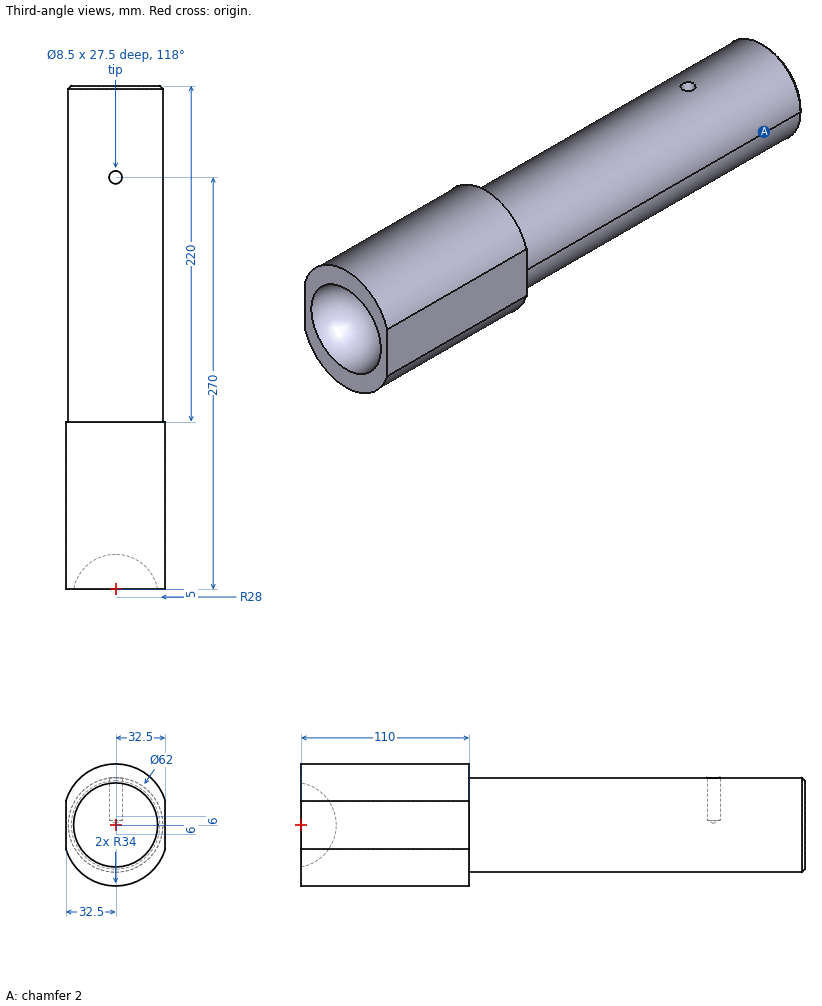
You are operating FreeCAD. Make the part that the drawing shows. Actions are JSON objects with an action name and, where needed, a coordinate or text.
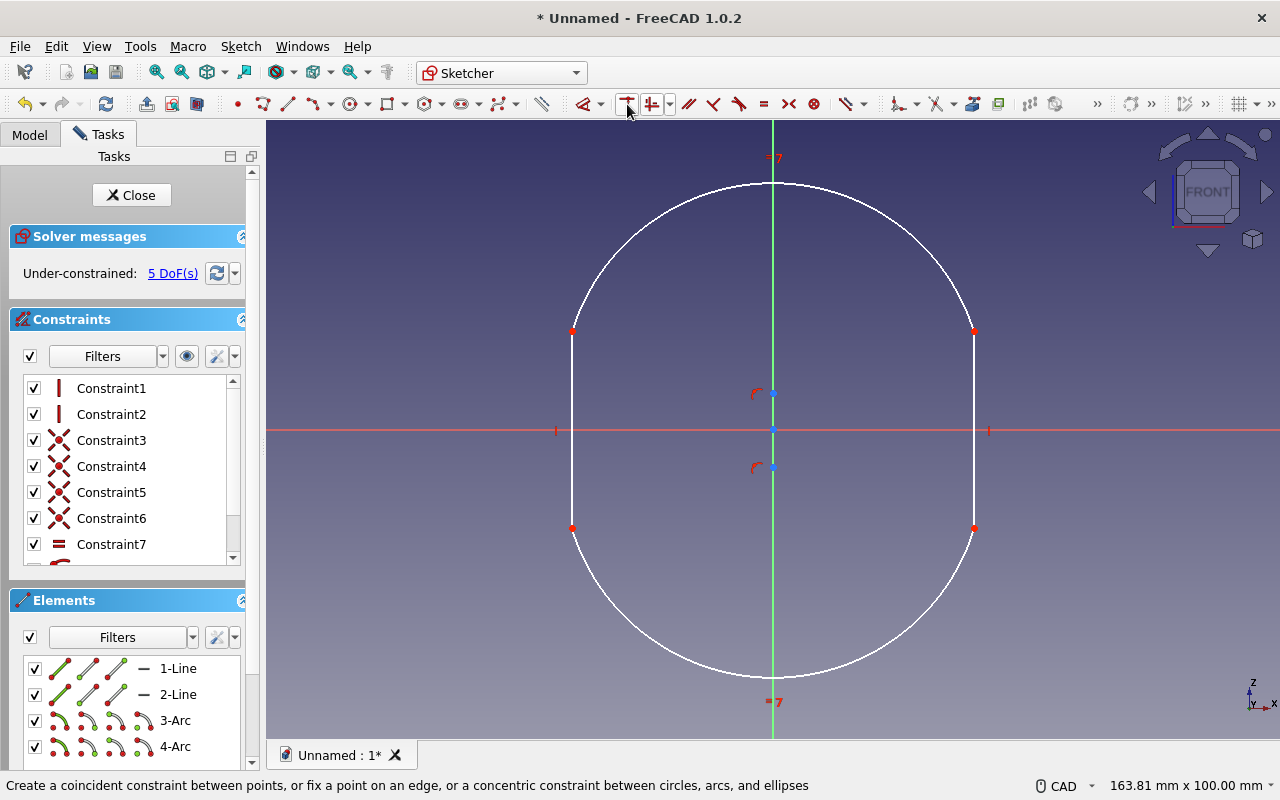
{"action": "left_click", "coordinate": [670, 651]}
{"action": "left_click", "coordinate": [654, 679]}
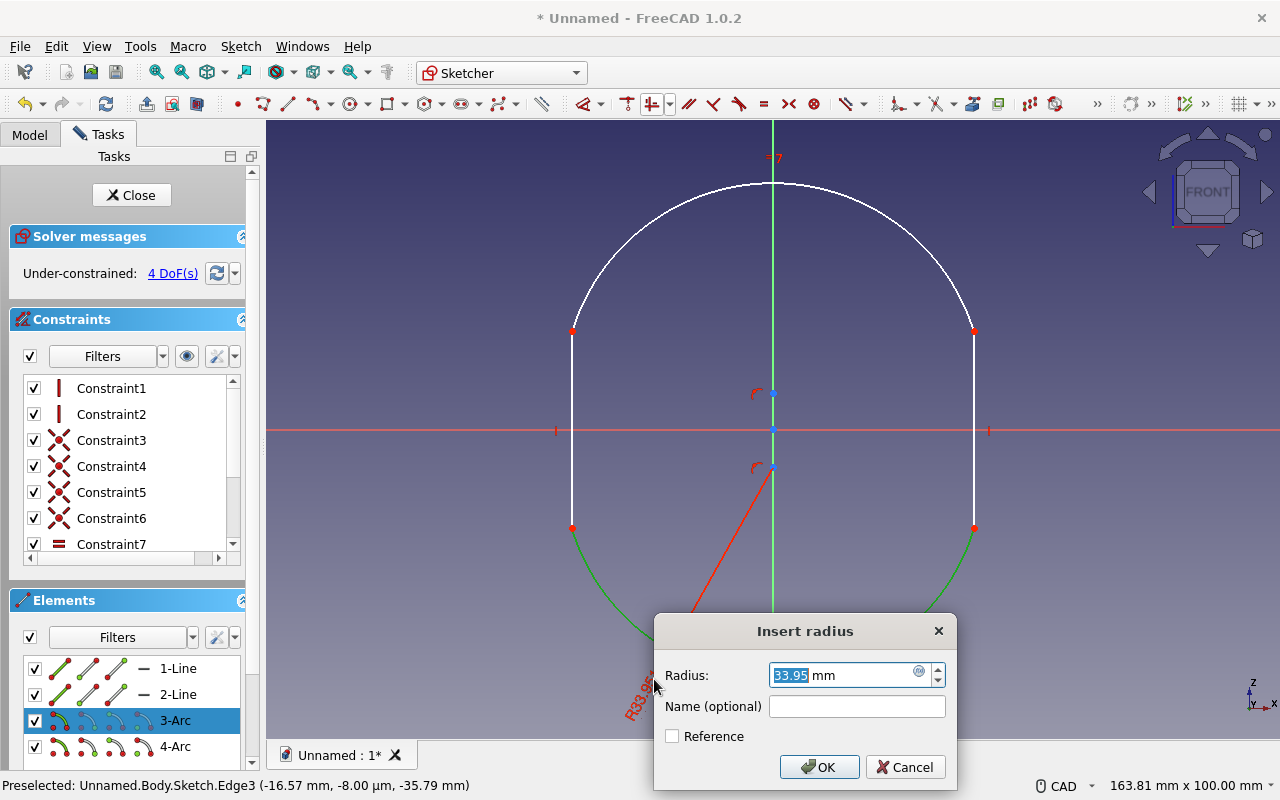
{"action": "type", "text": "34"}
{"action": "key", "text": "Return"}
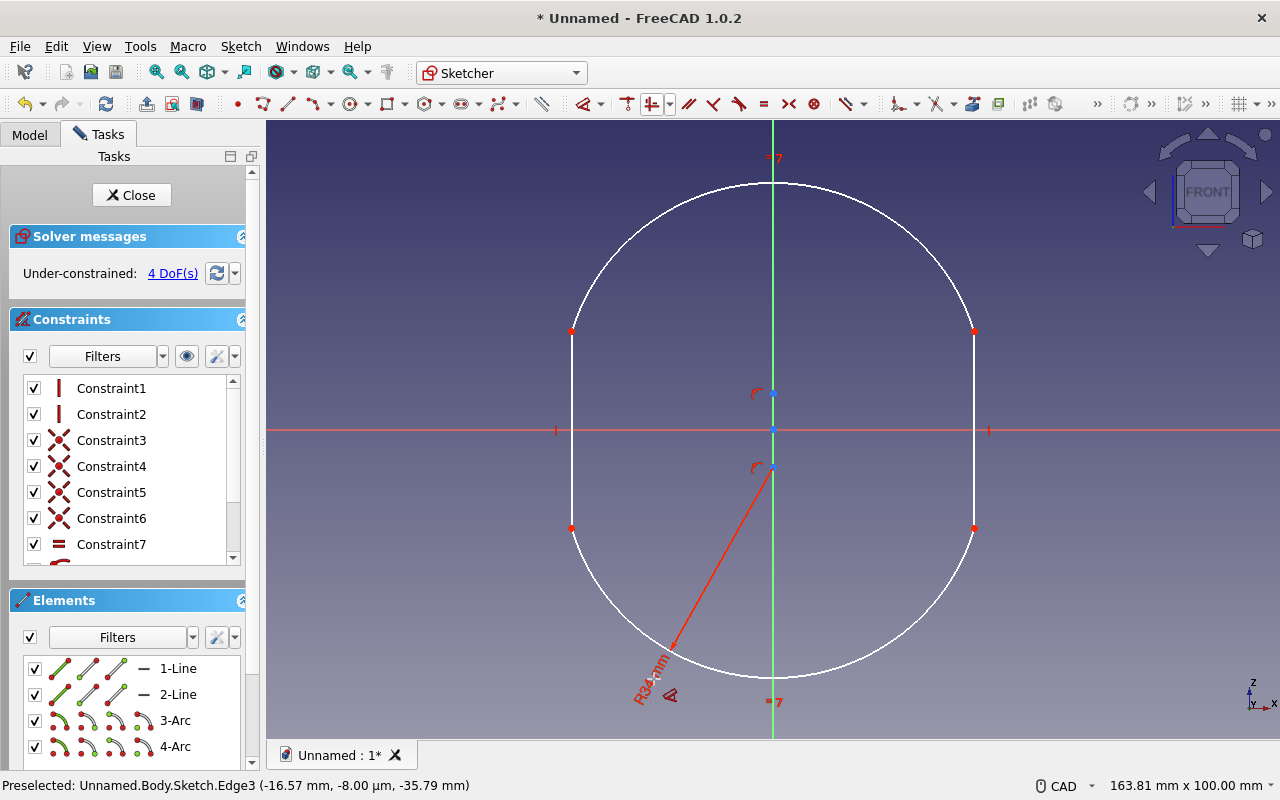
{"action": "left_click", "coordinate": [773, 468]}
{"action": "left_click", "coordinate": [807, 449]}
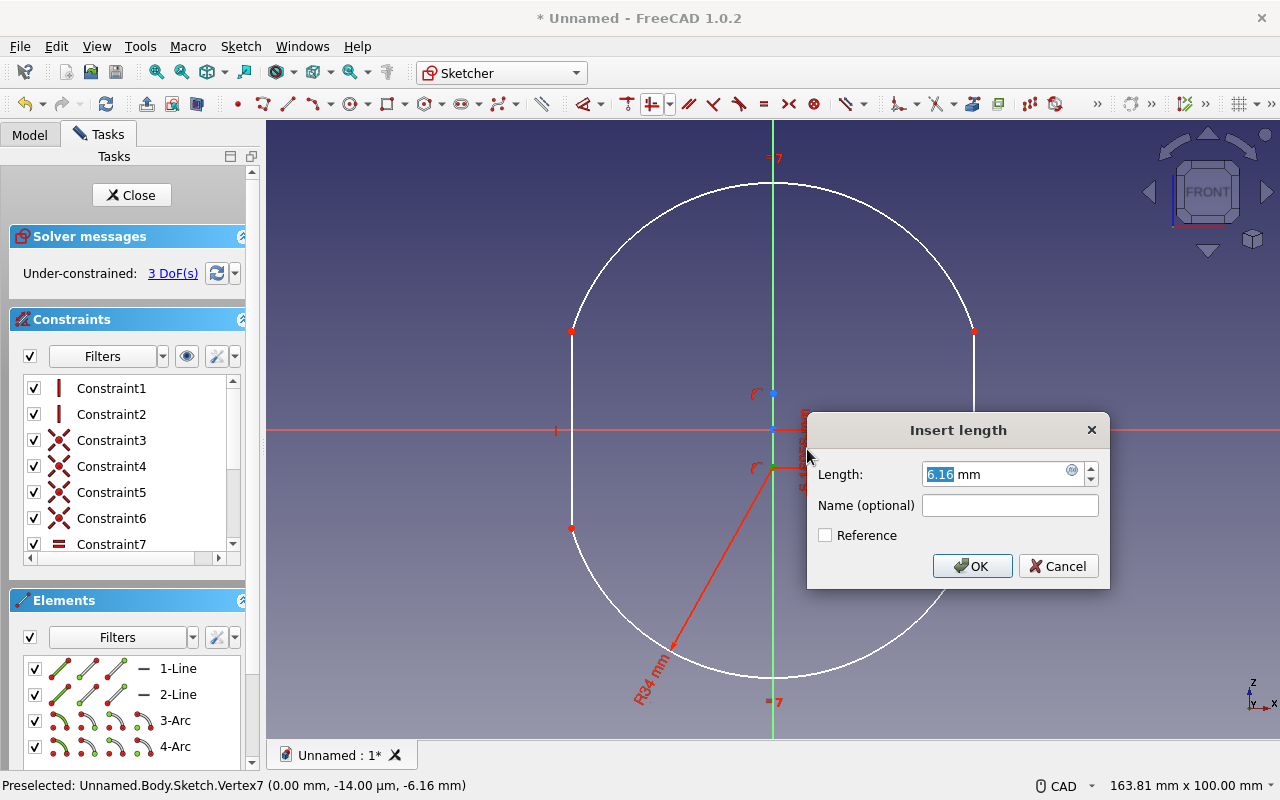
{"action": "type", "text": "6"}
{"action": "key", "text": "Return"}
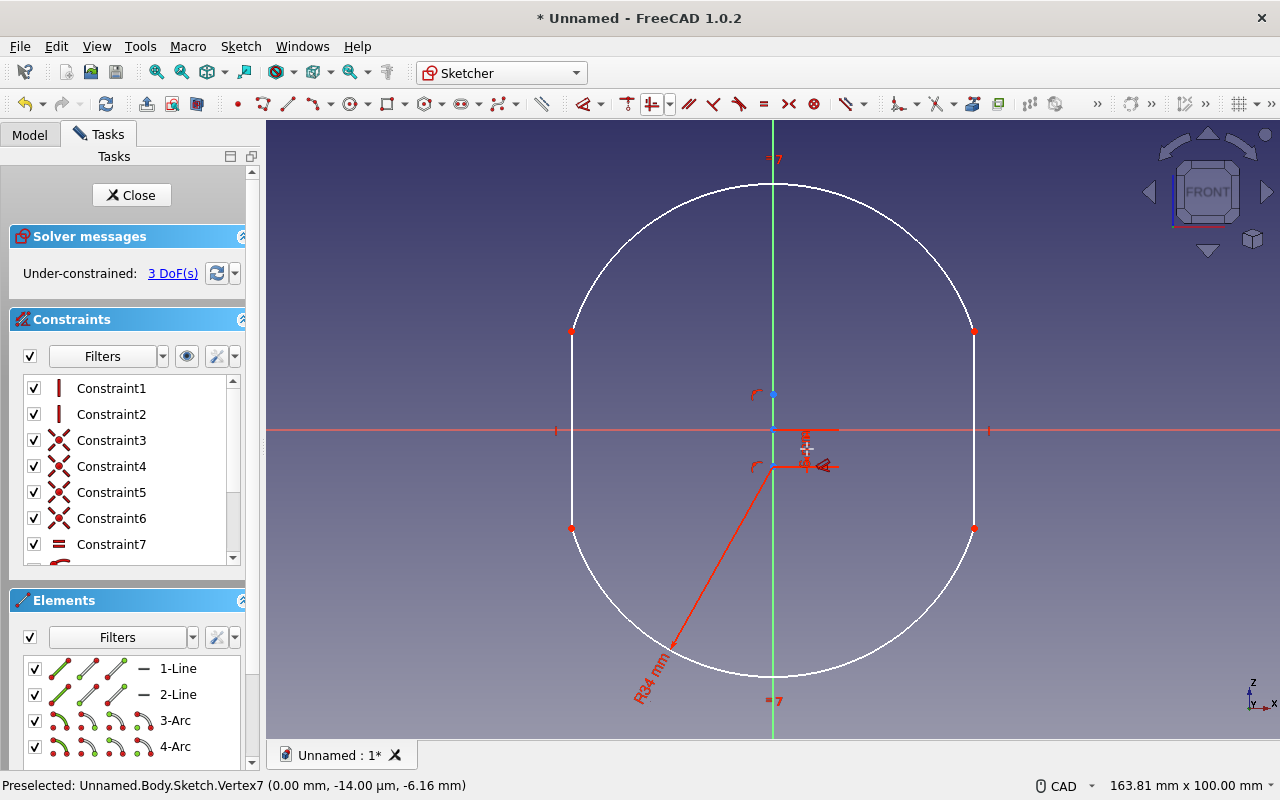
{"action": "left_click", "coordinate": [773, 394]}
{"action": "left_click", "coordinate": [807, 412]}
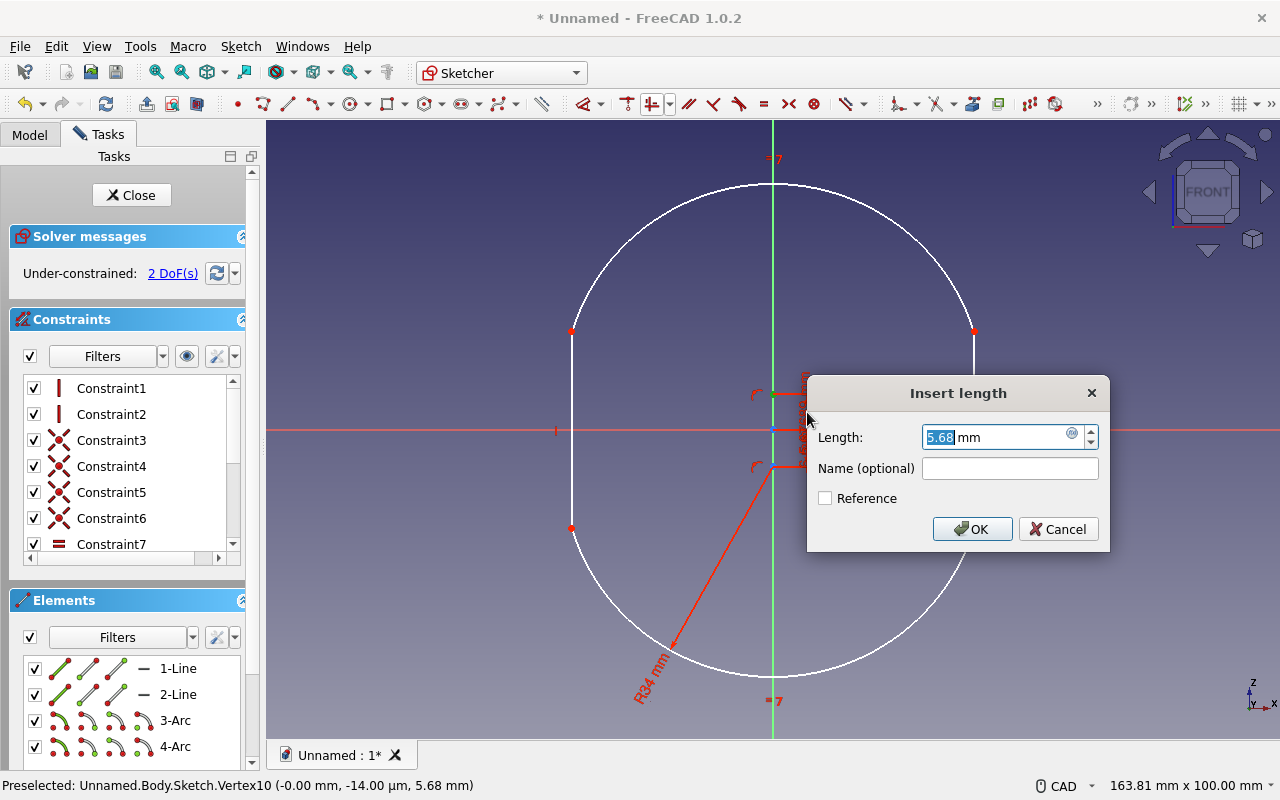
{"action": "type", "text": "6"}
{"action": "key", "text": "Return"}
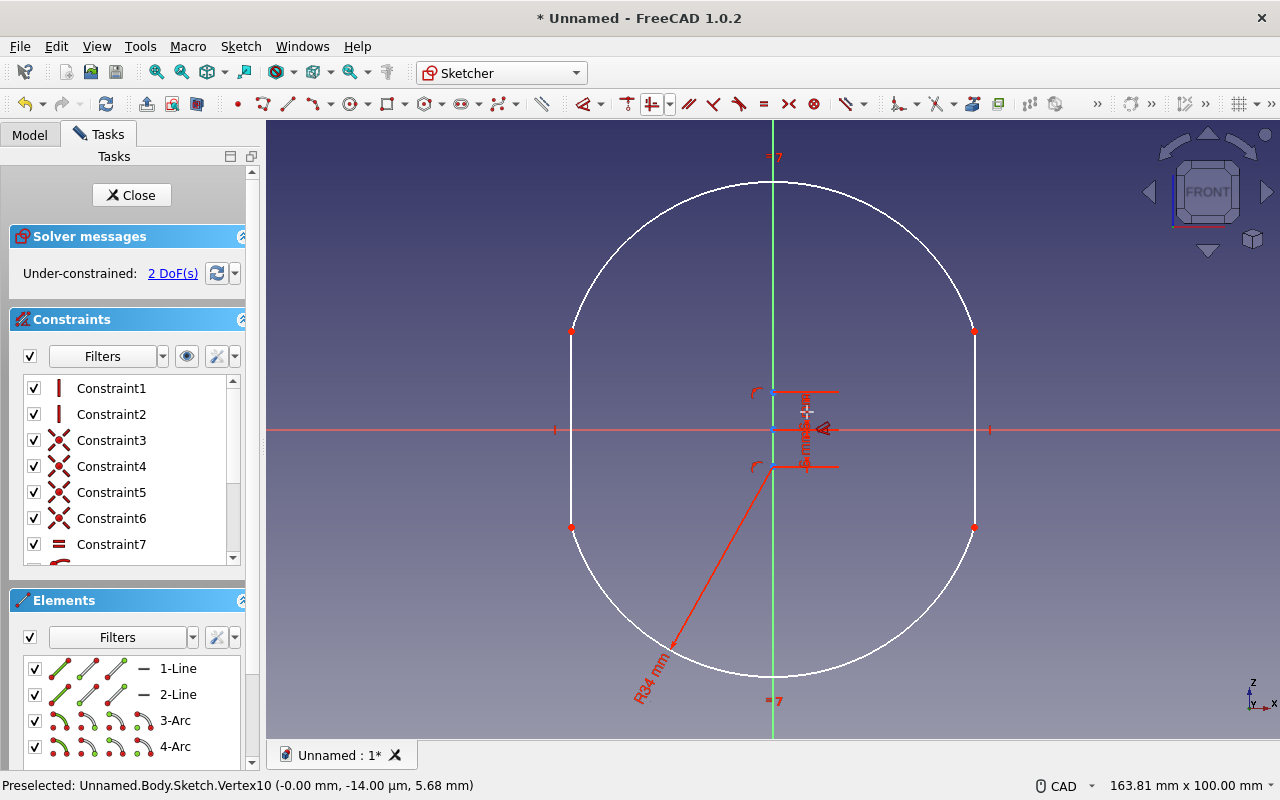
{"action": "left_click", "coordinate": [975, 332]}
{"action": "left_click", "coordinate": [874, 298]}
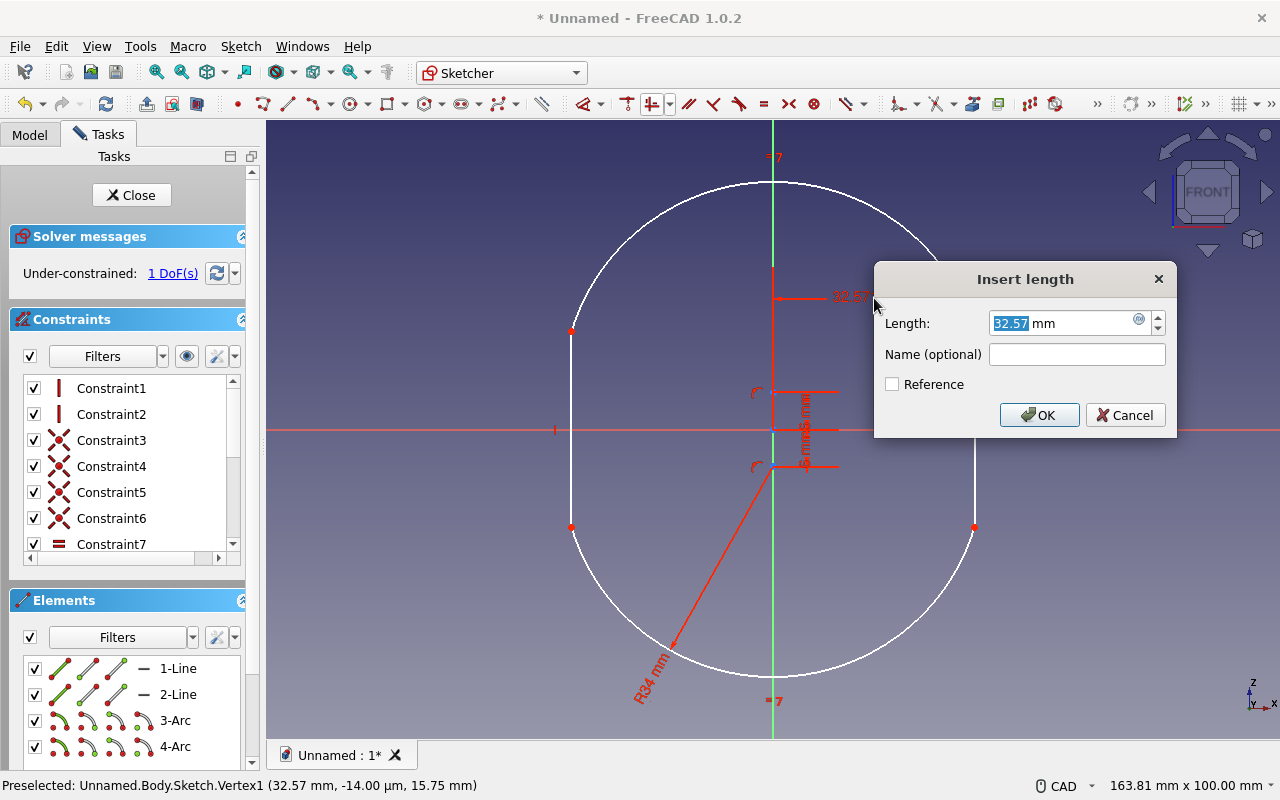
{"action": "type", "text": "32.5"}
{"action": "key", "text": "Return"}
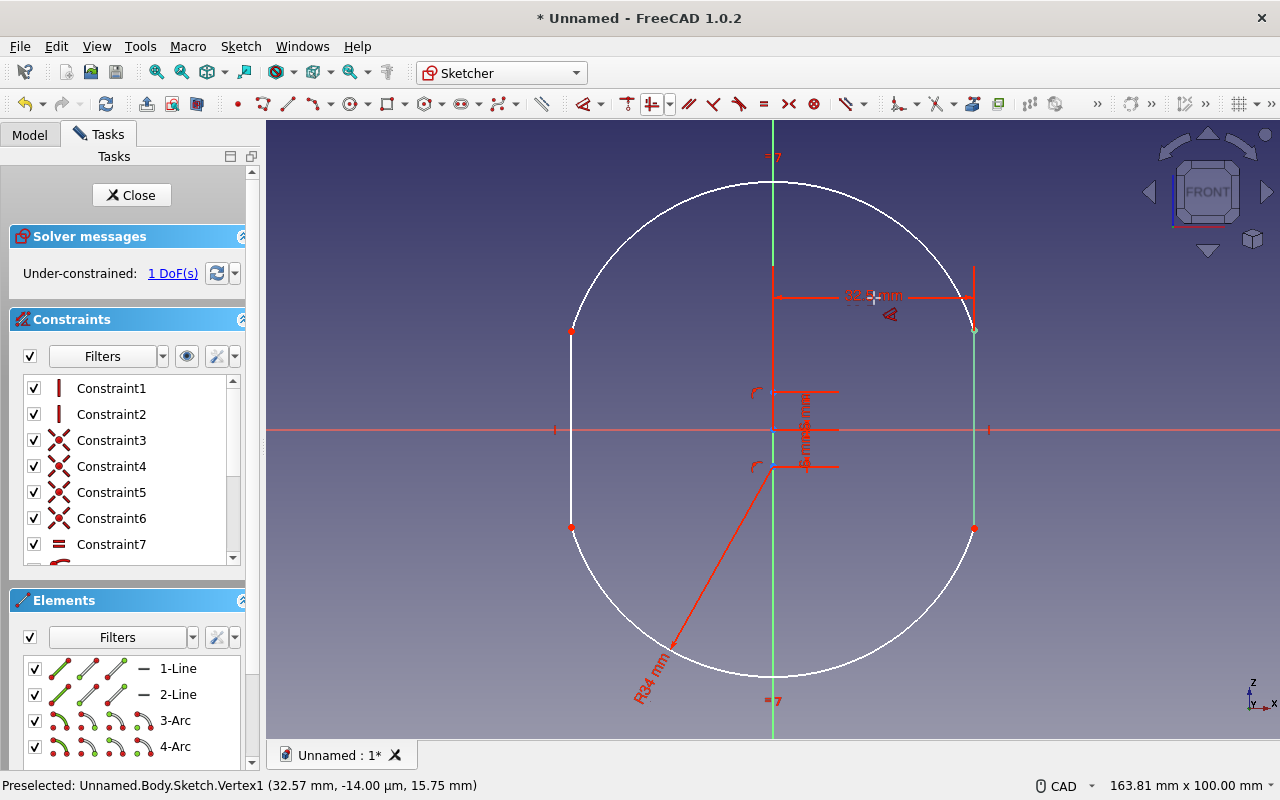
{"action": "left_click", "coordinate": [571, 527]}
{"action": "left_click", "coordinate": [672, 561]}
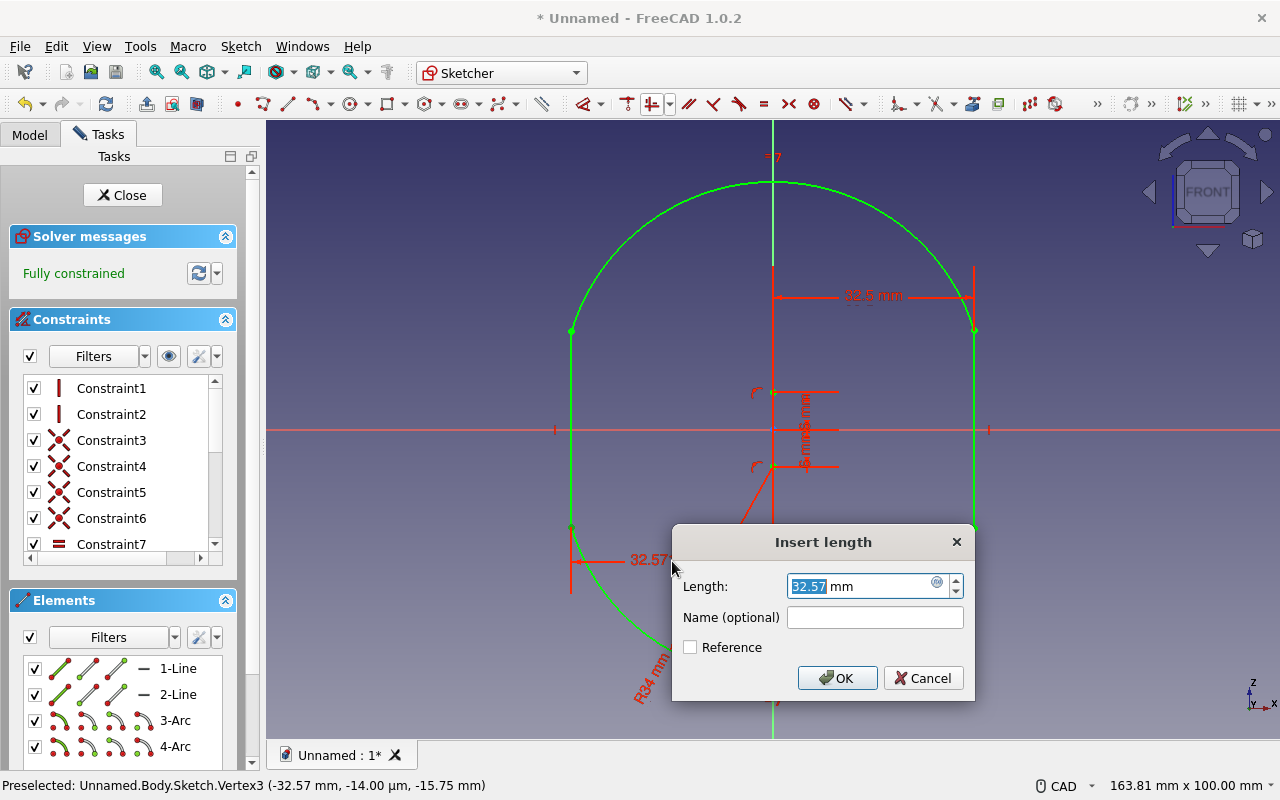
{"action": "type", "text": "32.5"}
{"action": "key", "text": "Return"}
{"action": "key", "text": "Escape"}